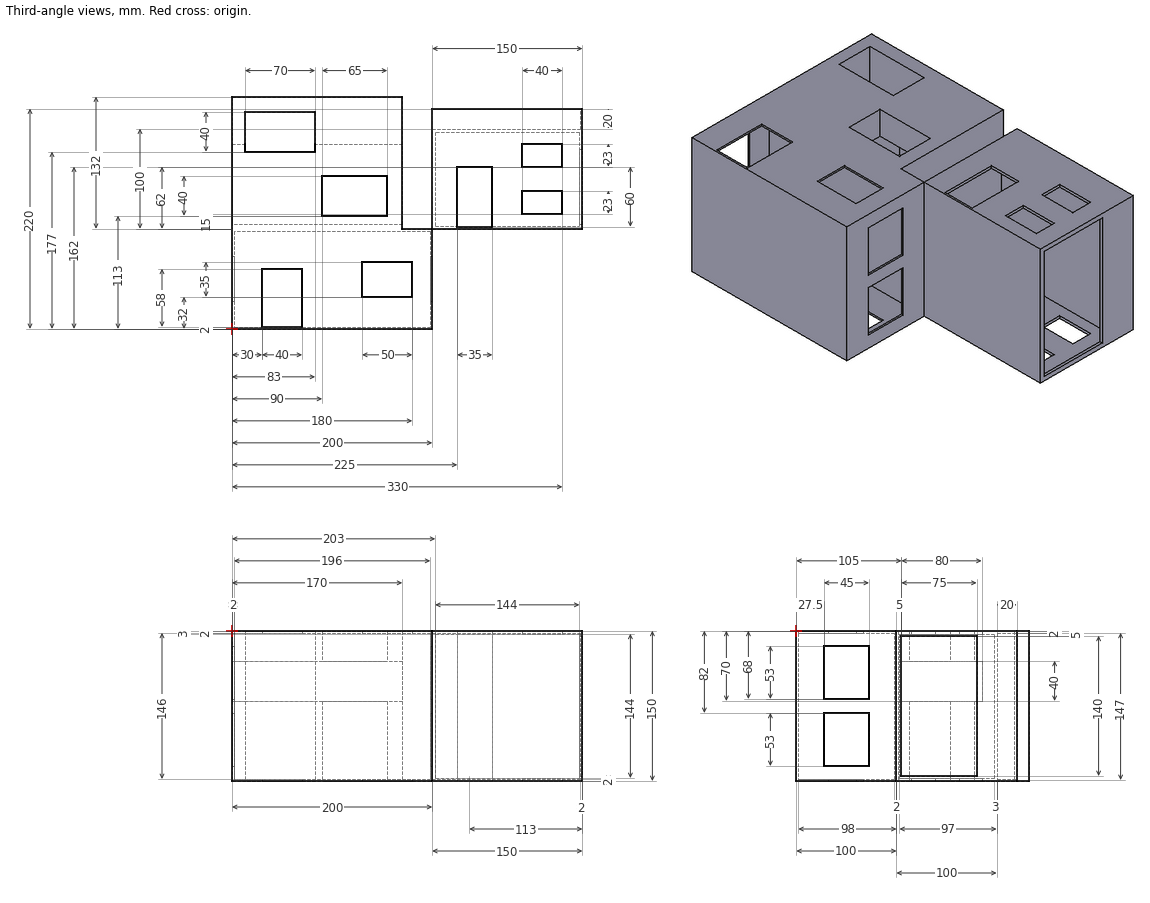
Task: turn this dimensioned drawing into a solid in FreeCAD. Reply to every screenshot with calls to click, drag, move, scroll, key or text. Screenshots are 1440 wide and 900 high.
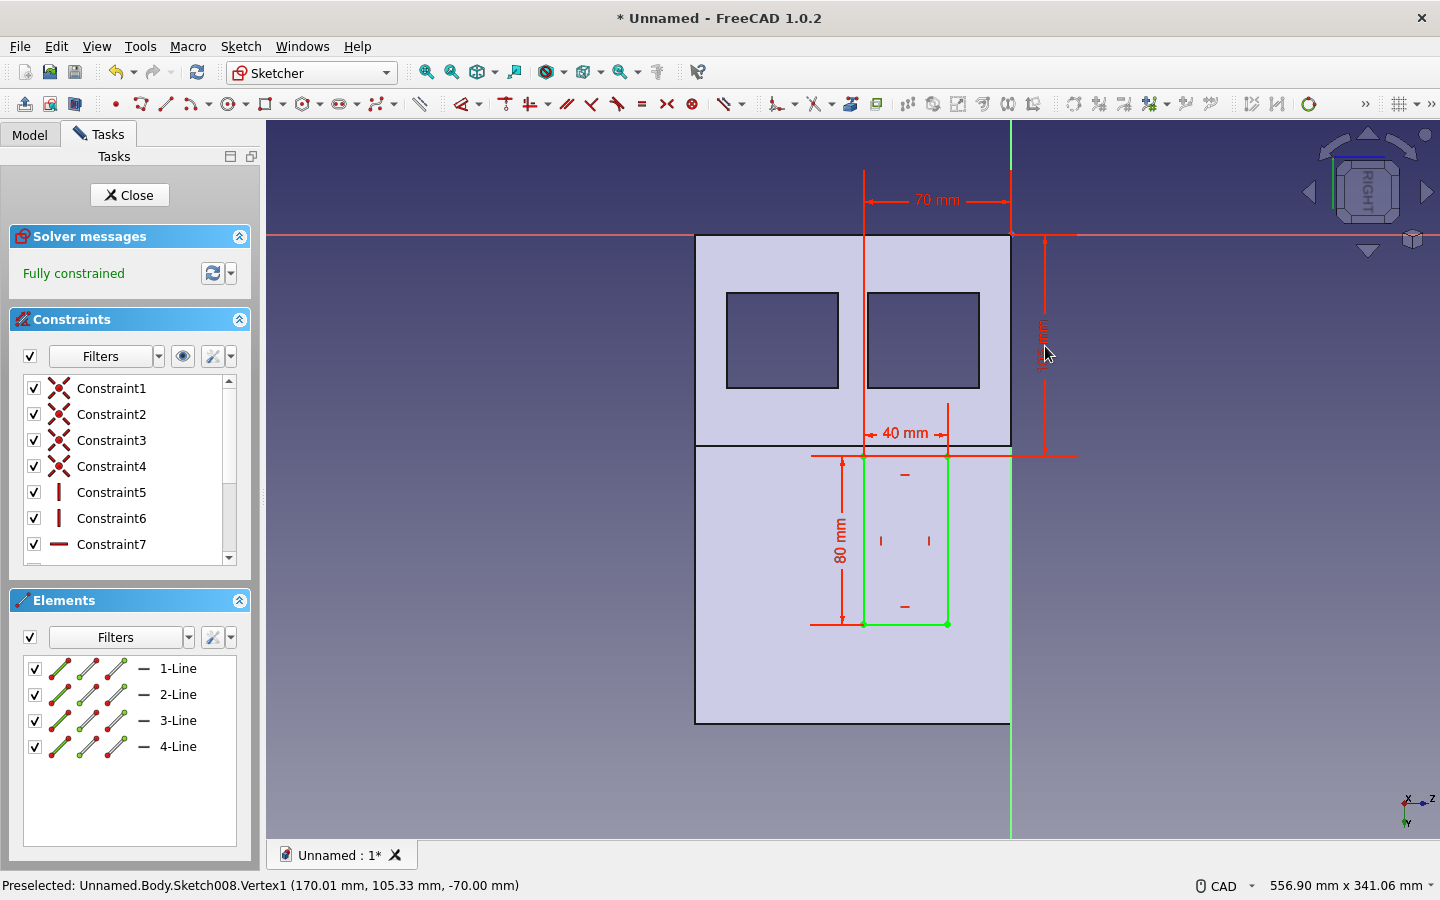
click(130, 195)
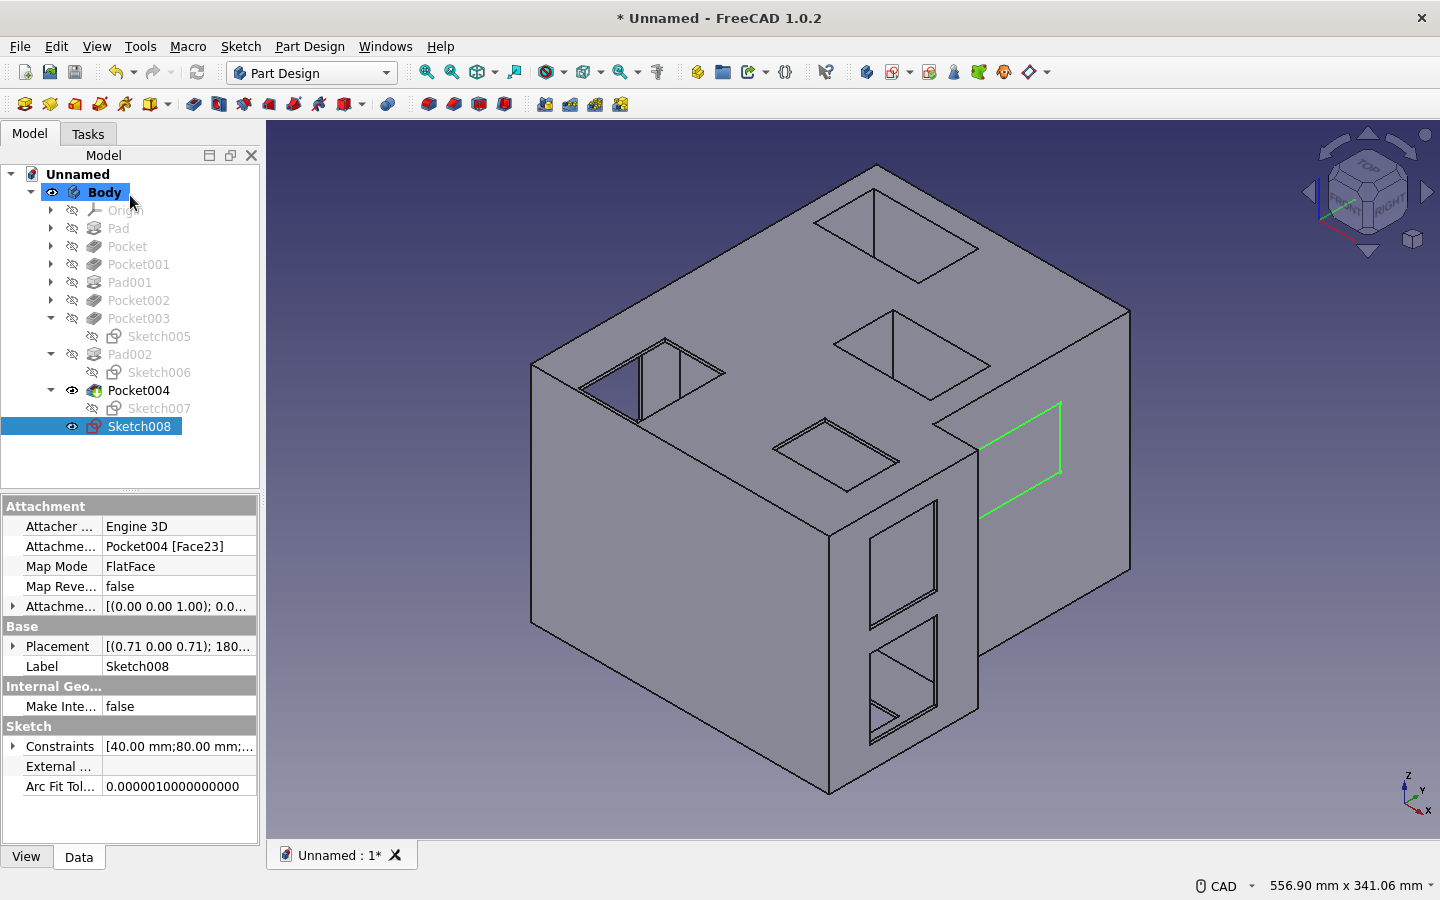
click(194, 104)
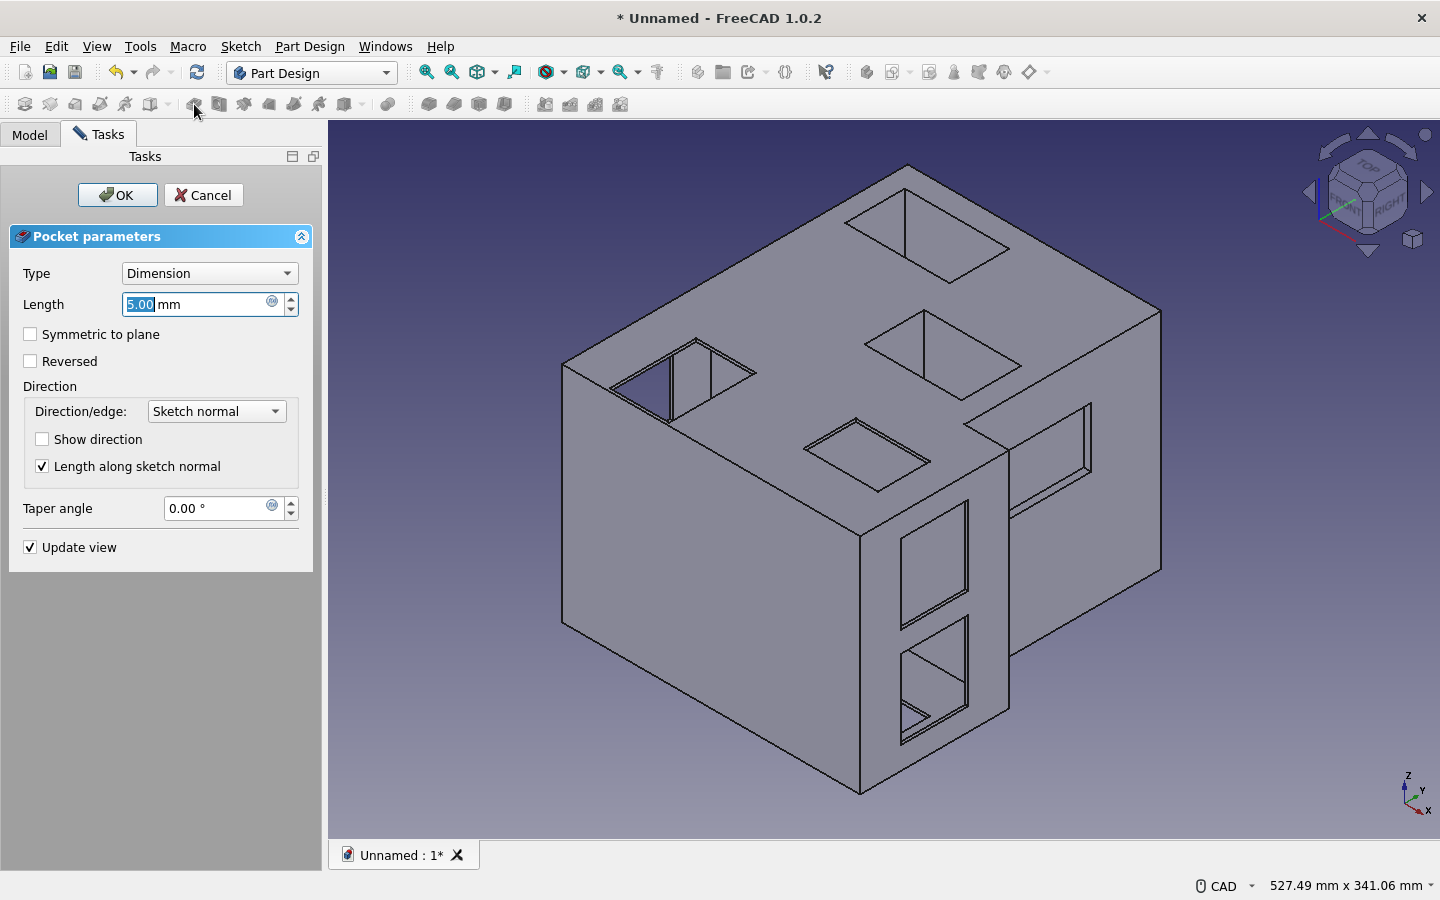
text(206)
key(Tab)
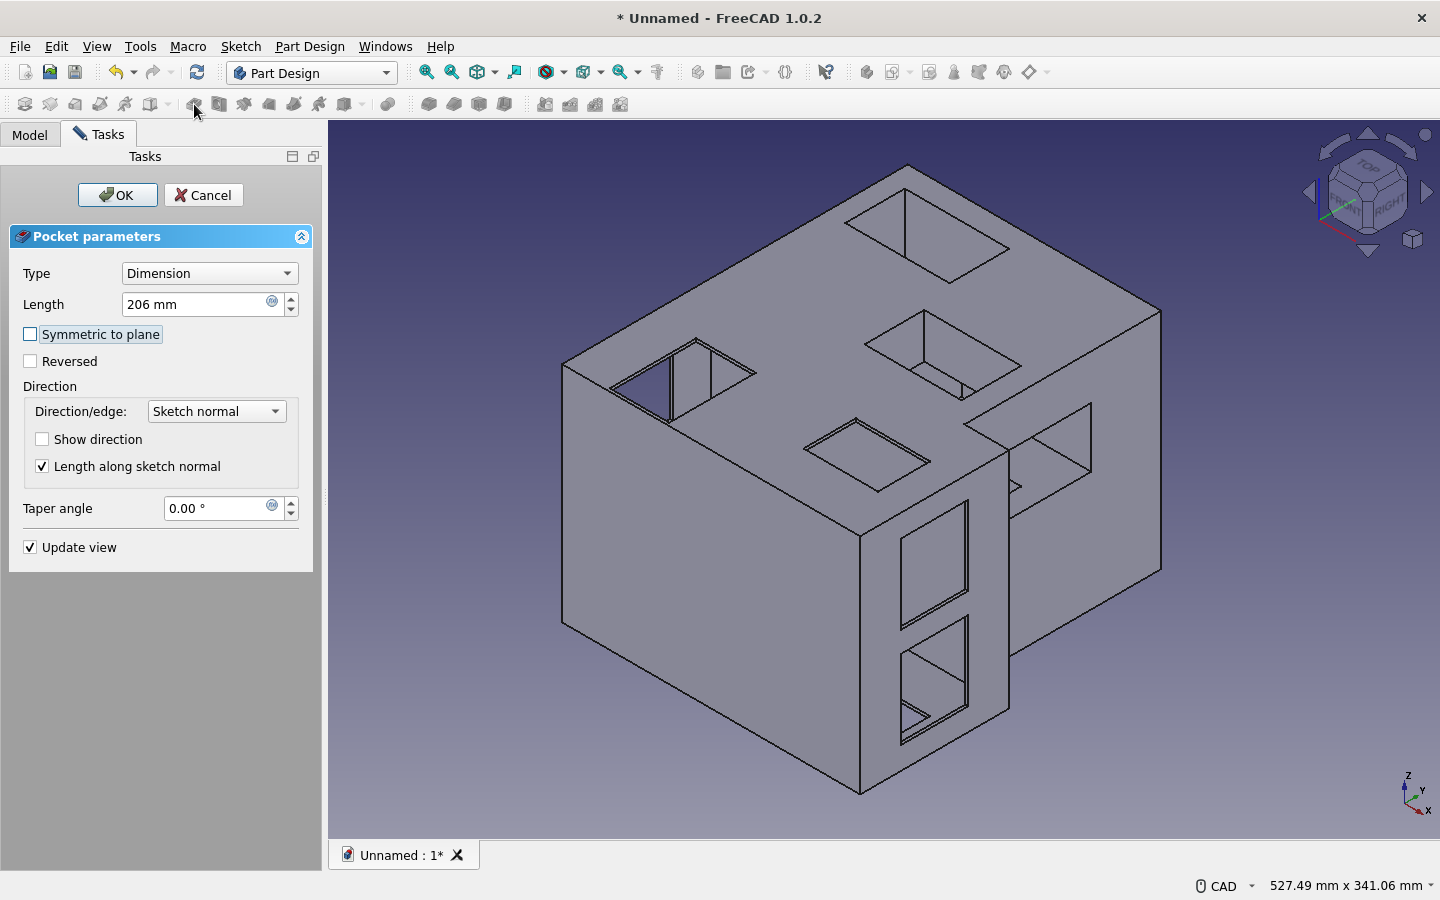
click(118, 195)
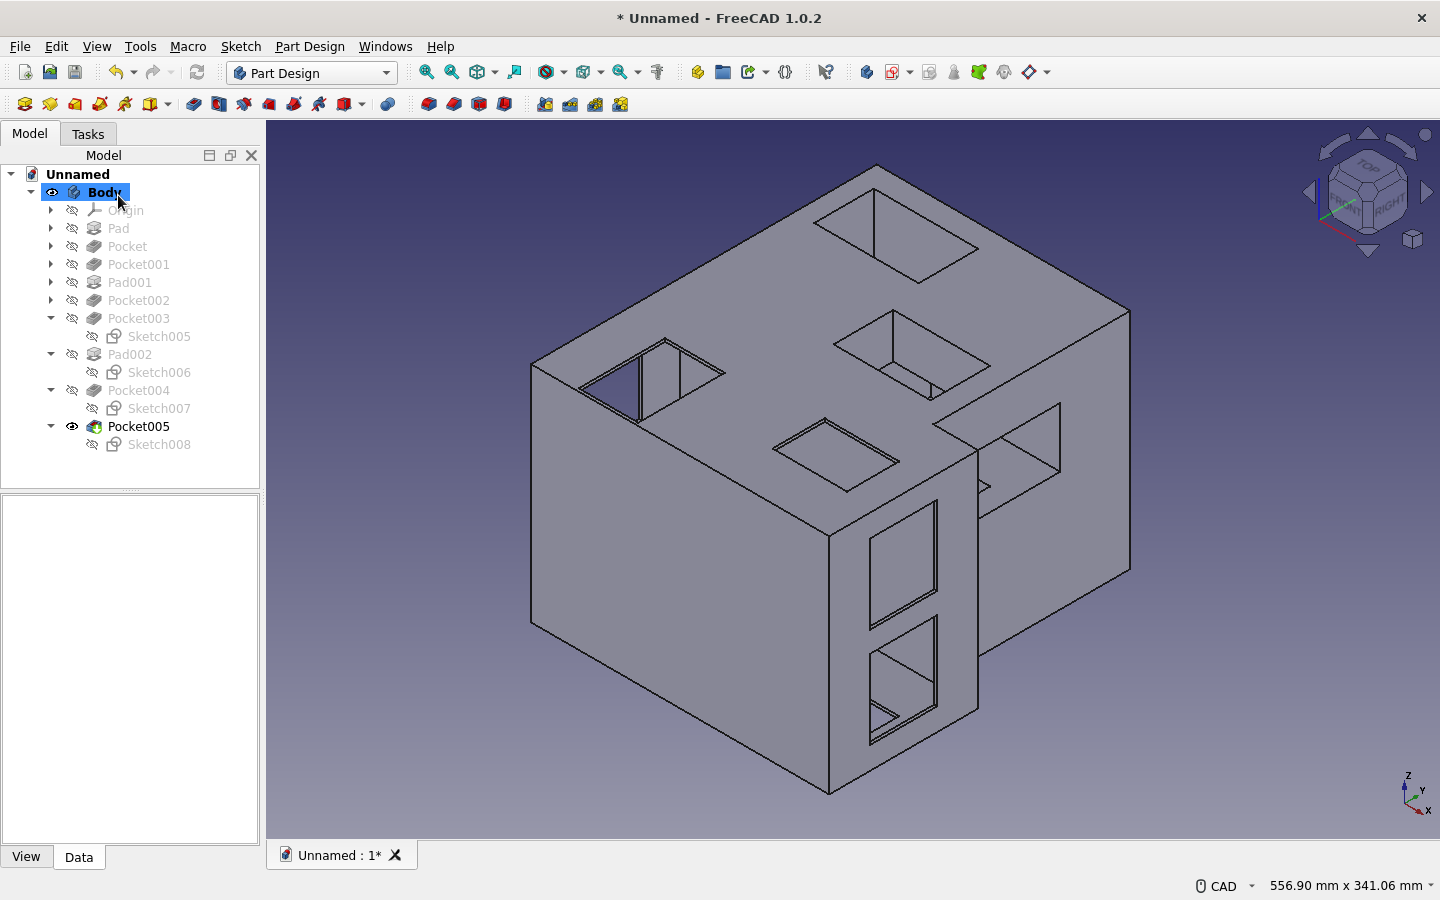
click(867, 72)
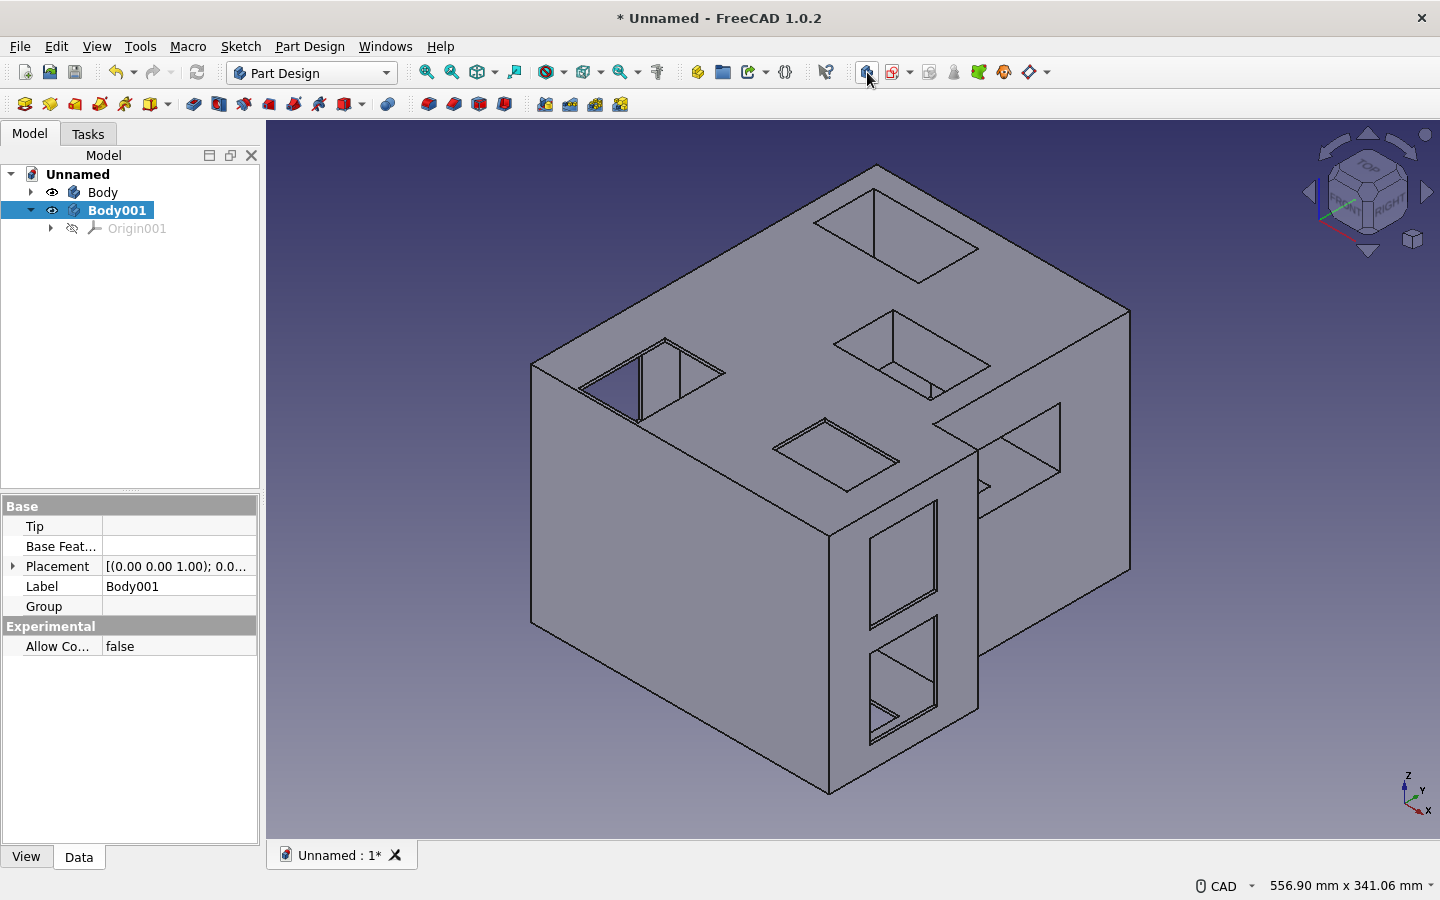
click(51, 228)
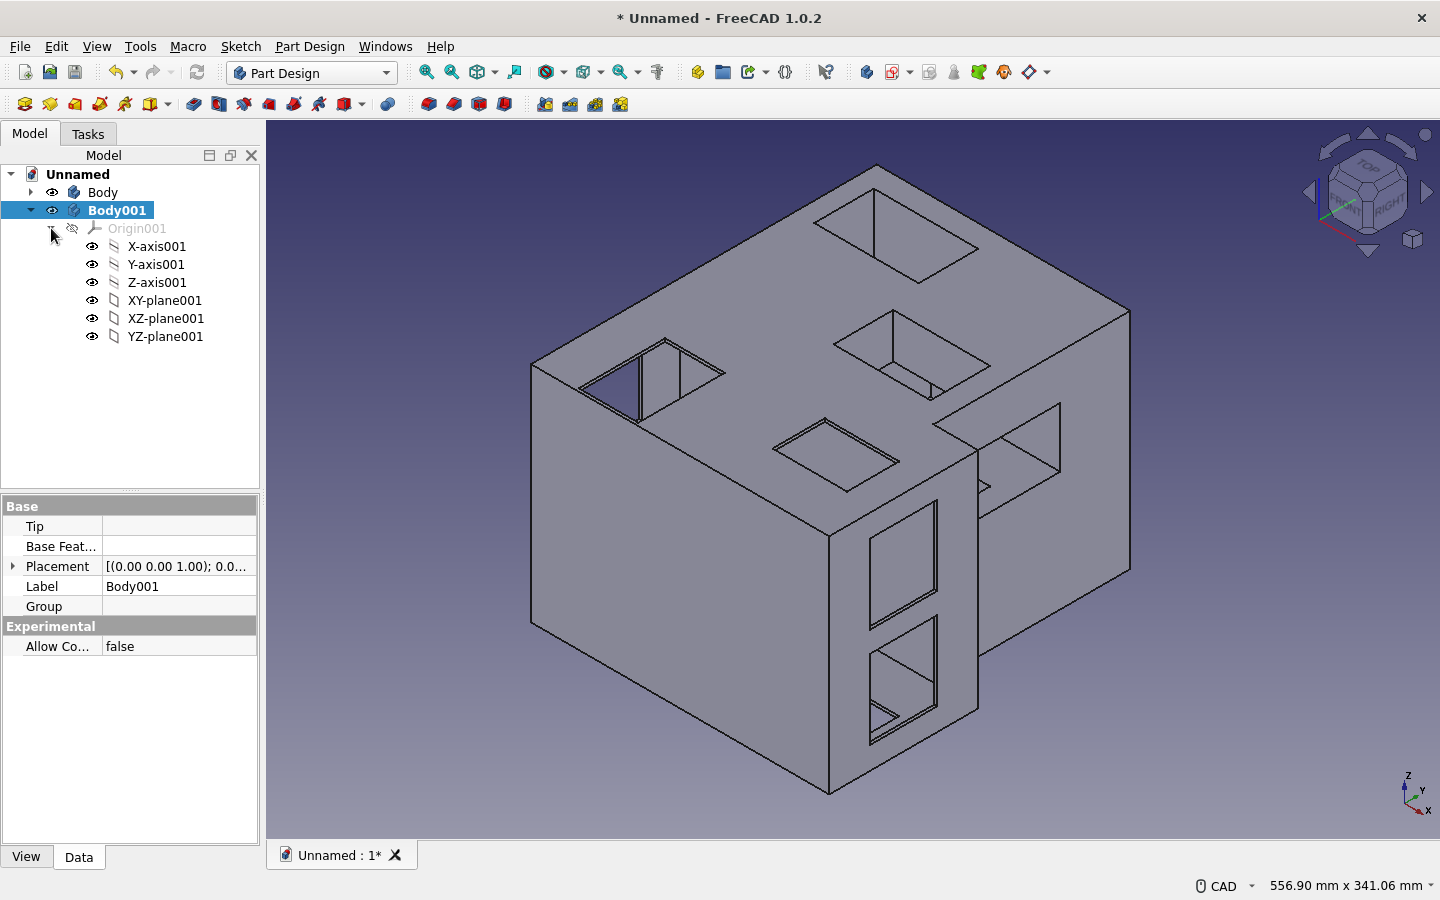
click(137, 318)